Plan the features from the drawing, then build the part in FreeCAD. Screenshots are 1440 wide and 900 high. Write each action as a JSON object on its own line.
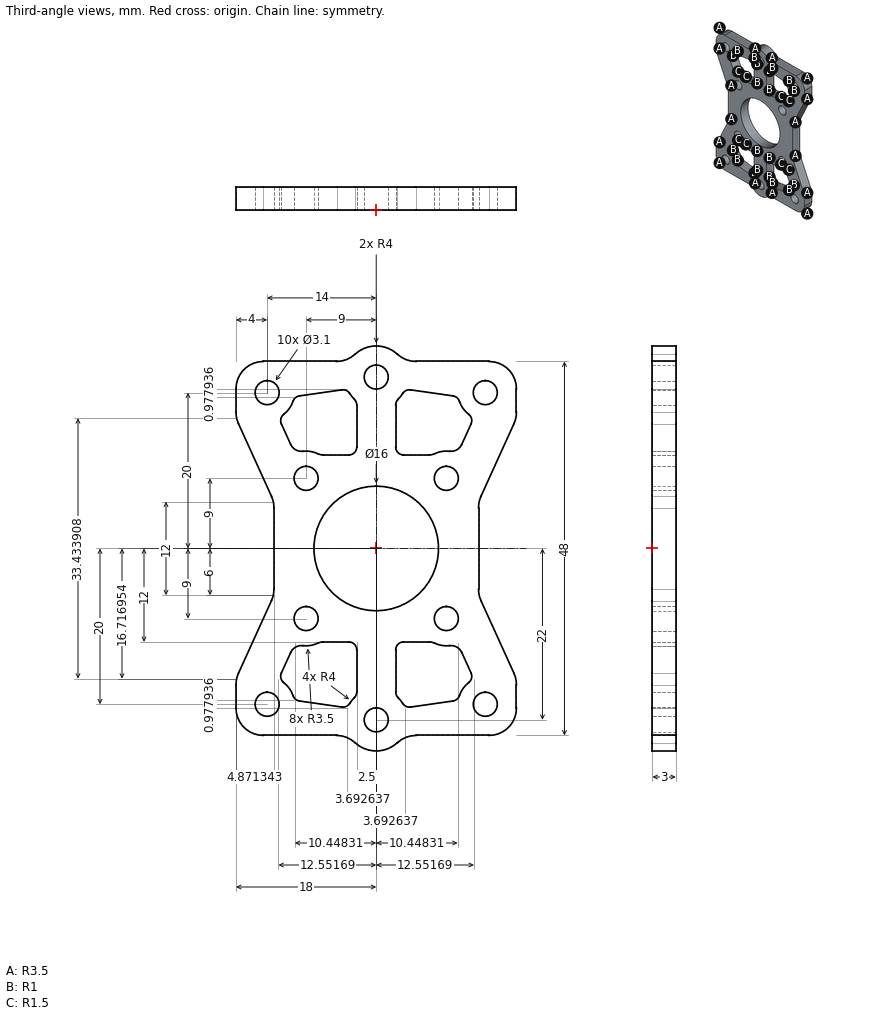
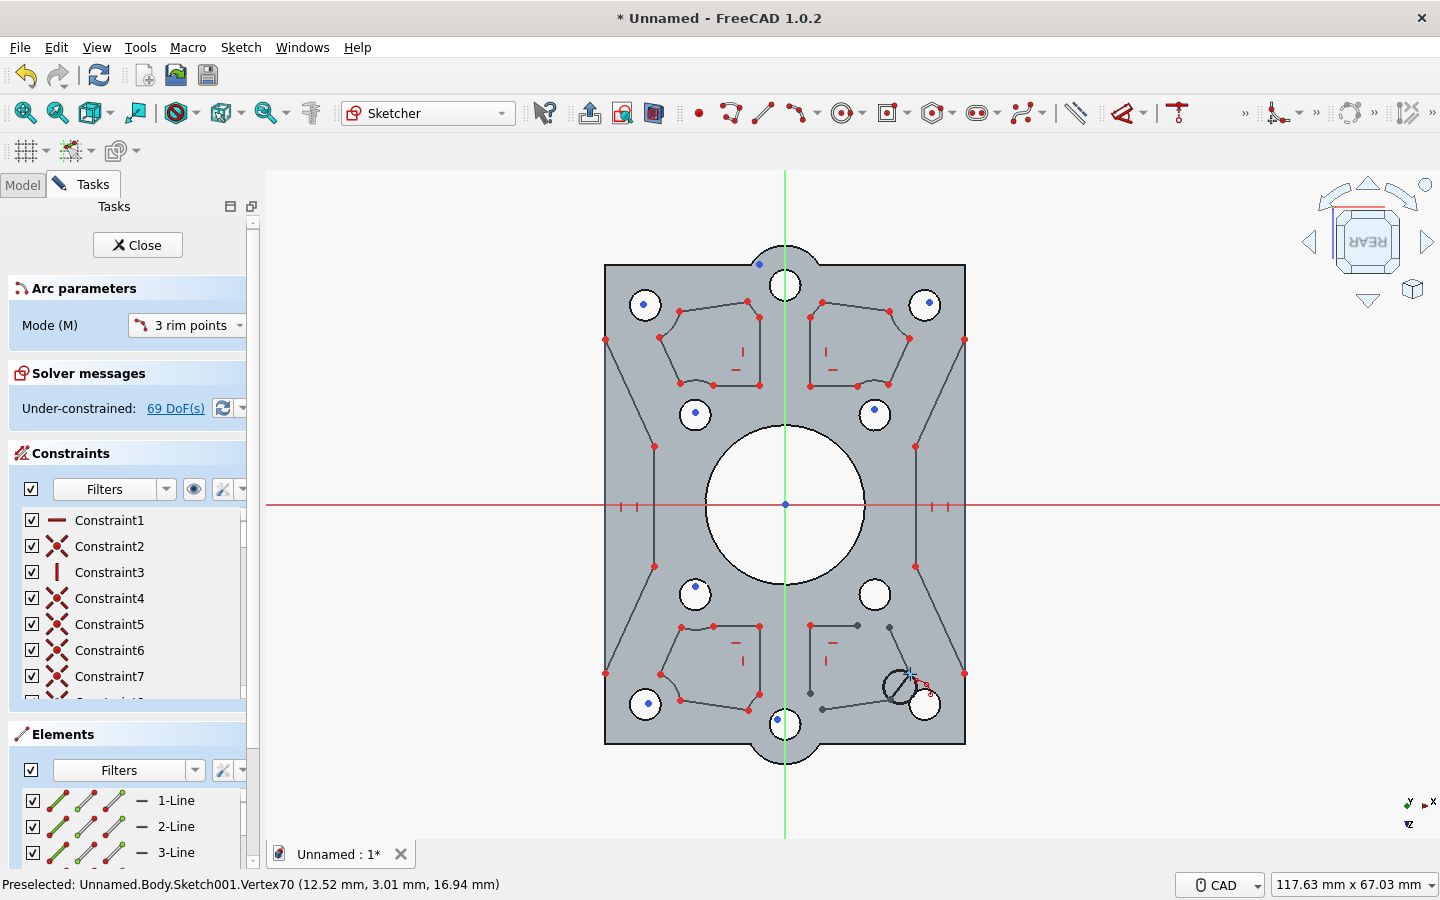
{"action": "scroll", "coordinate": [897, 684], "scroll_direction": "up", "scroll_amount": 7}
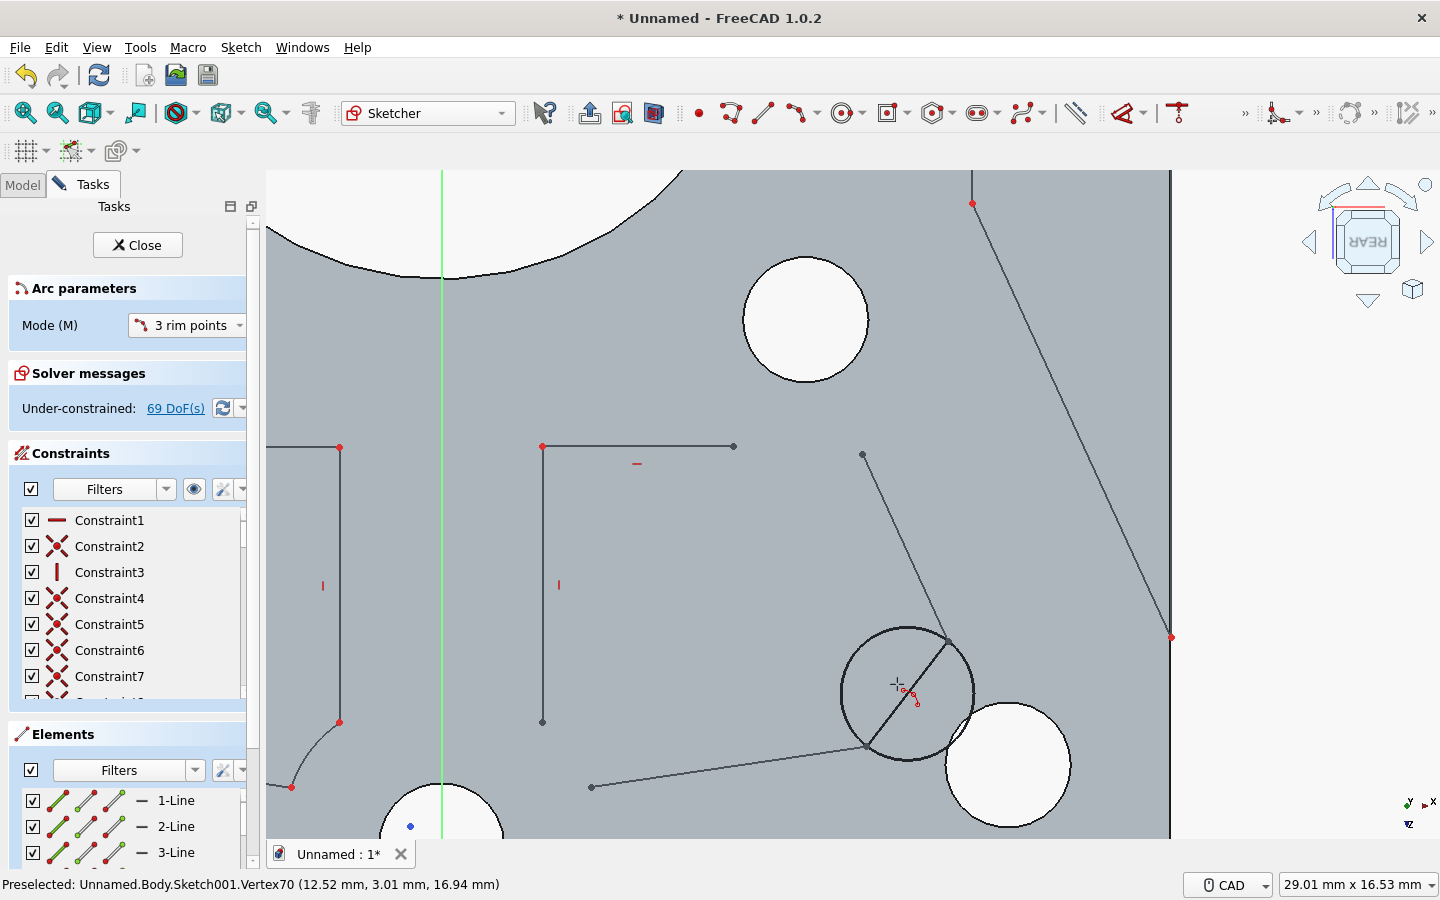
{"action": "left_click", "coordinate": [895, 680]}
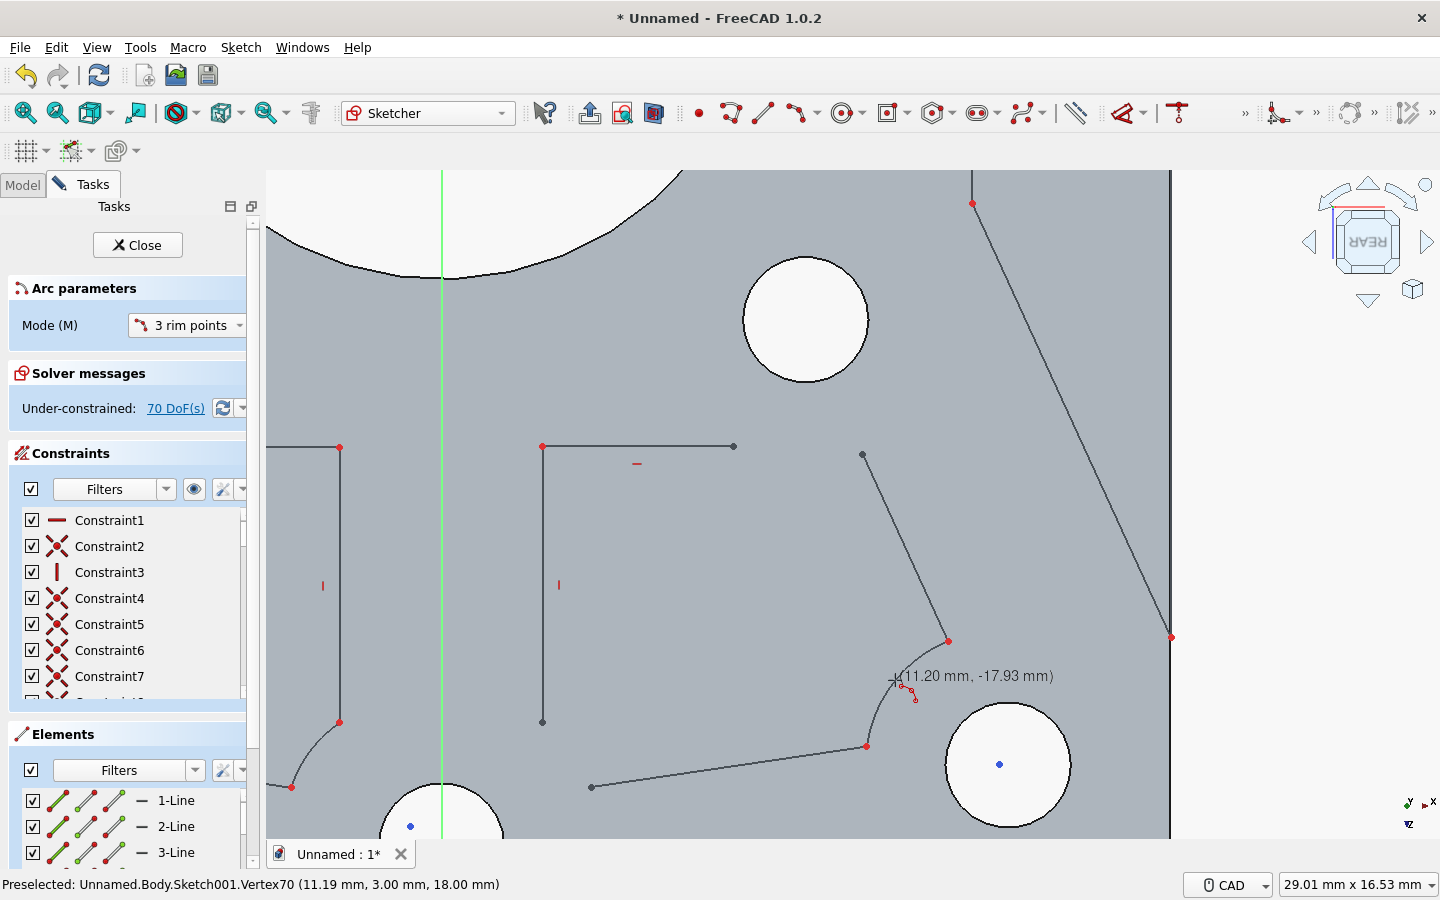
{"action": "scroll", "coordinate": [897, 684], "scroll_direction": "down", "scroll_amount": 7}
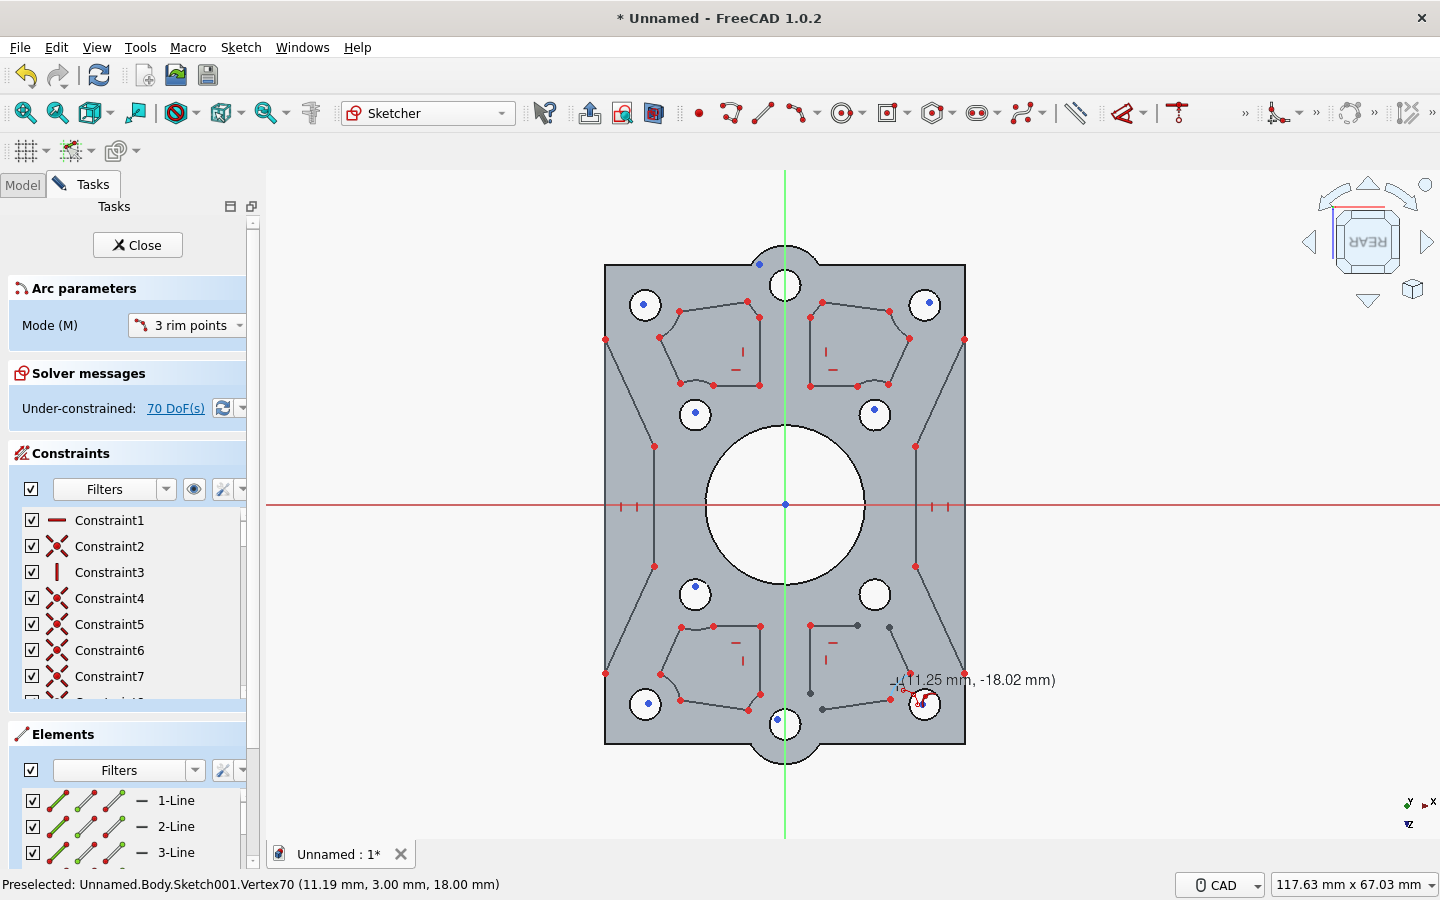
{"action": "left_click", "coordinate": [889, 628]}
{"action": "left_click", "coordinate": [857, 626]}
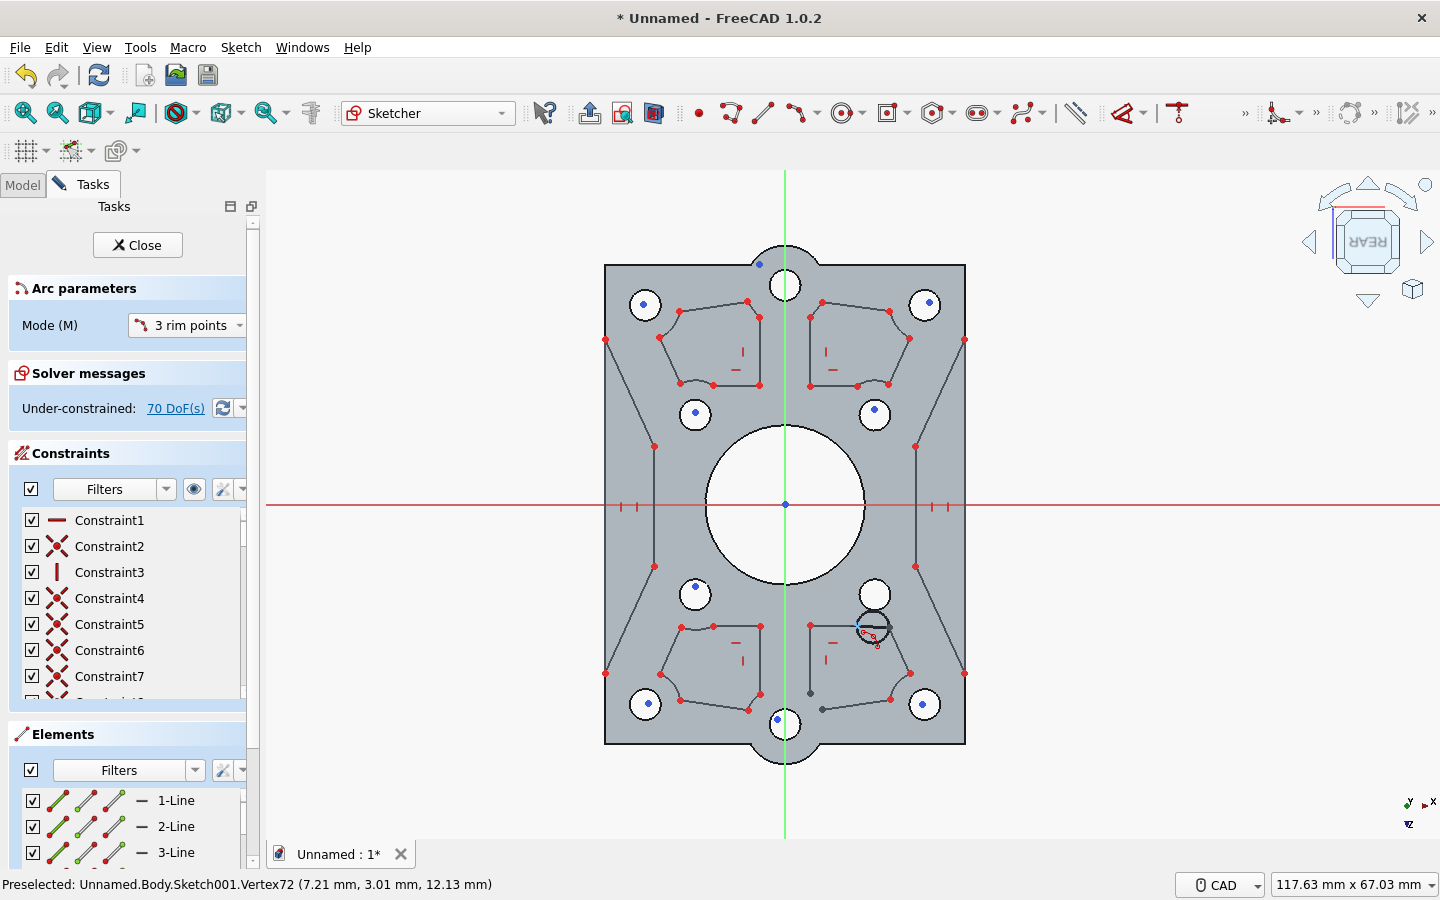
{"action": "scroll", "coordinate": [873, 630], "scroll_direction": "up", "scroll_amount": 7}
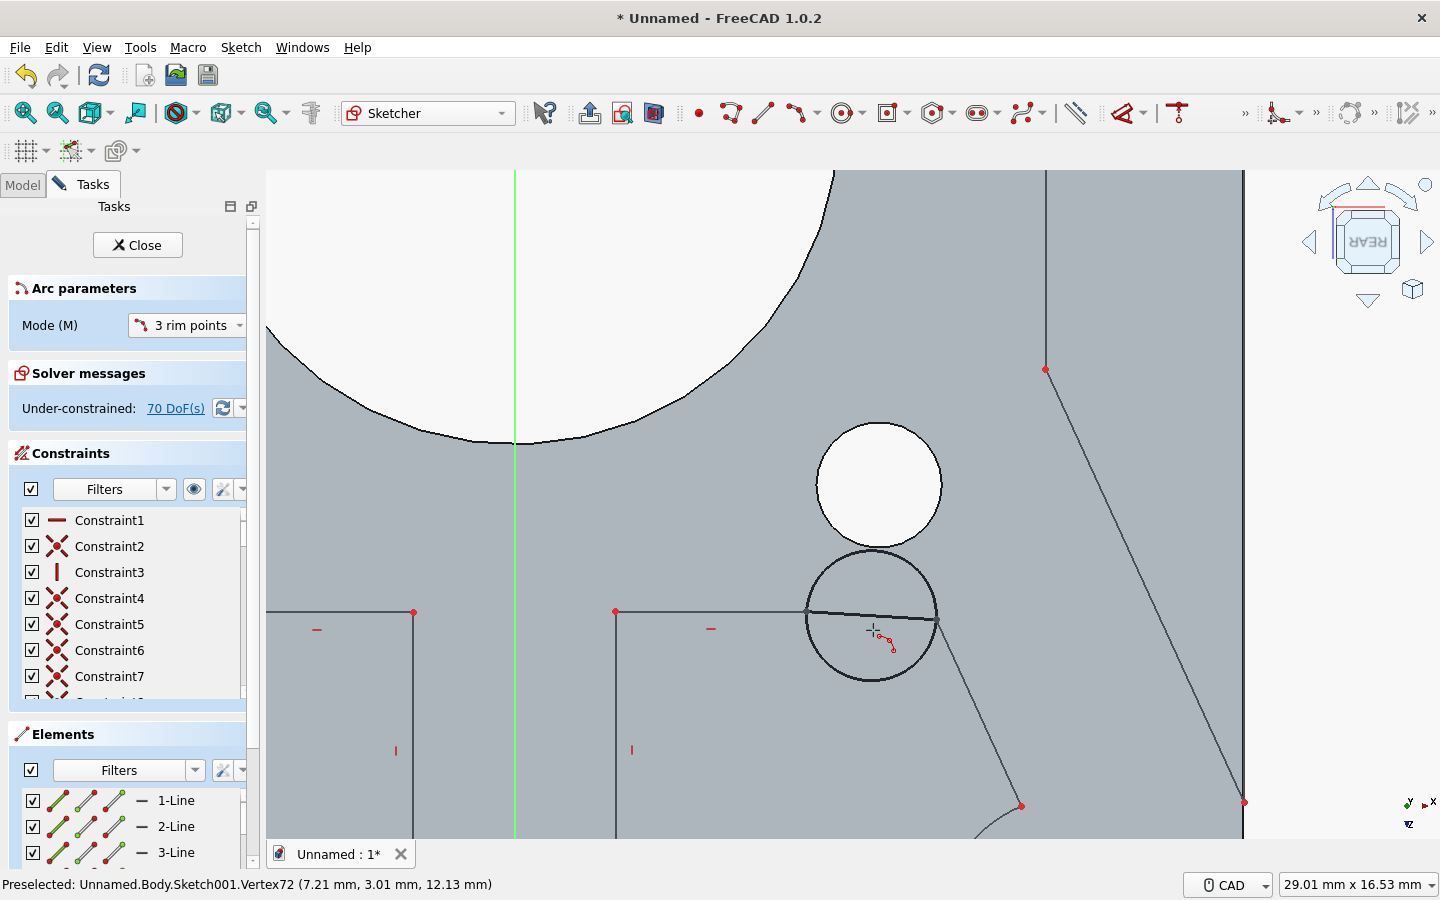
{"action": "left_click", "coordinate": [871, 626]}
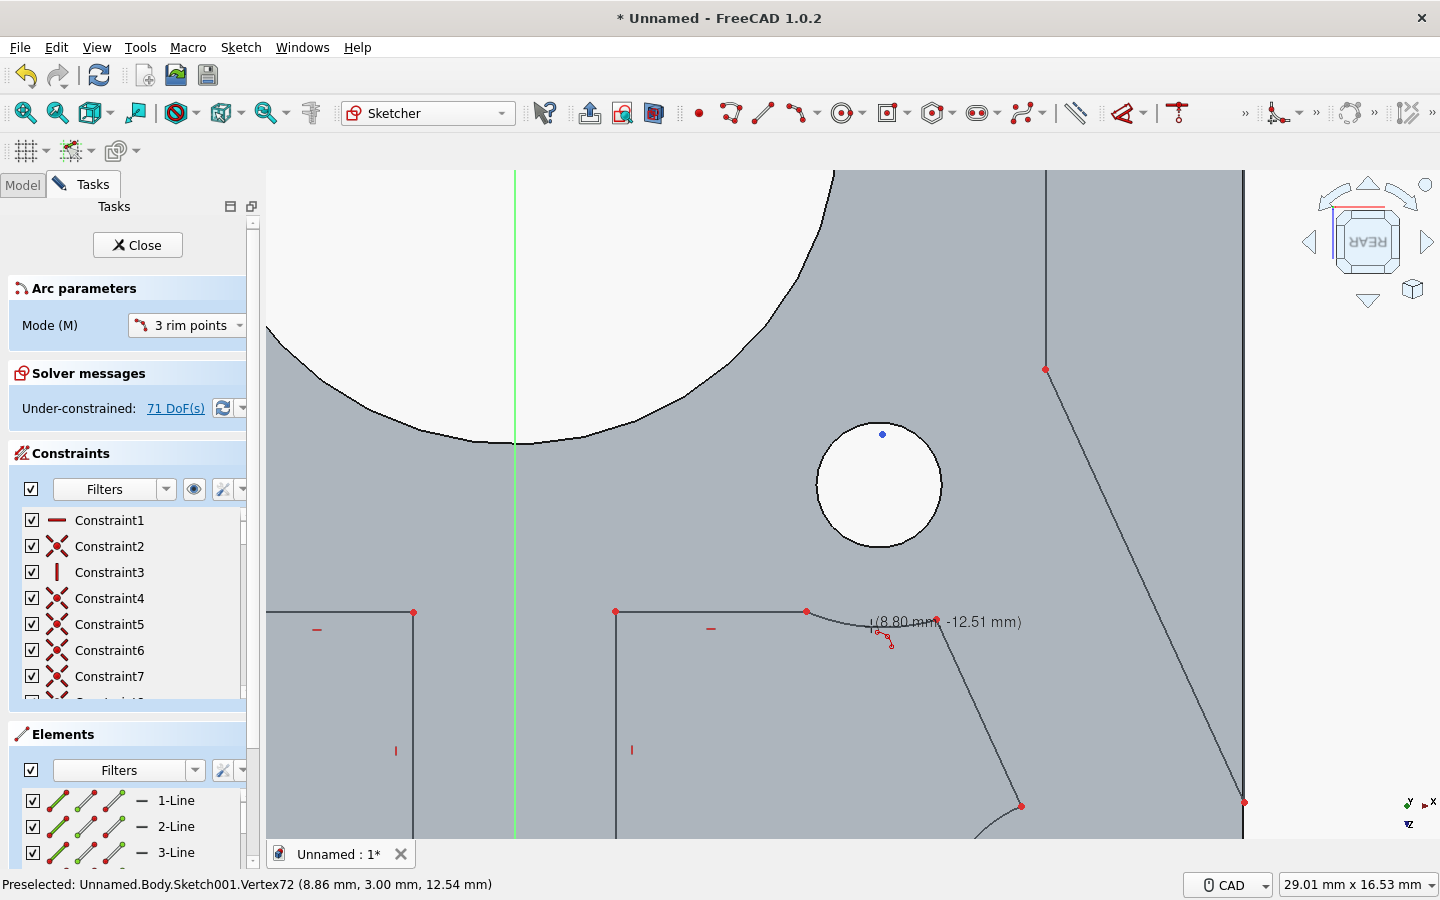
{"action": "scroll", "coordinate": [873, 630], "scroll_direction": "down", "scroll_amount": 7}